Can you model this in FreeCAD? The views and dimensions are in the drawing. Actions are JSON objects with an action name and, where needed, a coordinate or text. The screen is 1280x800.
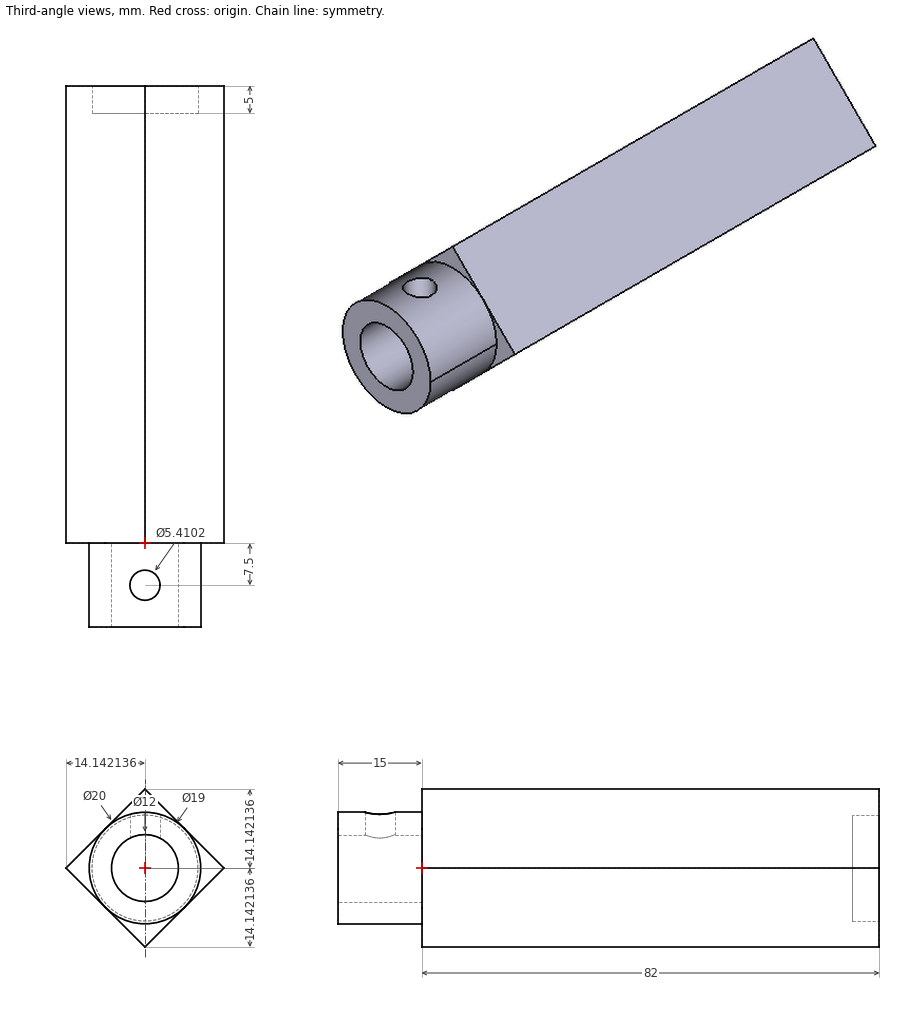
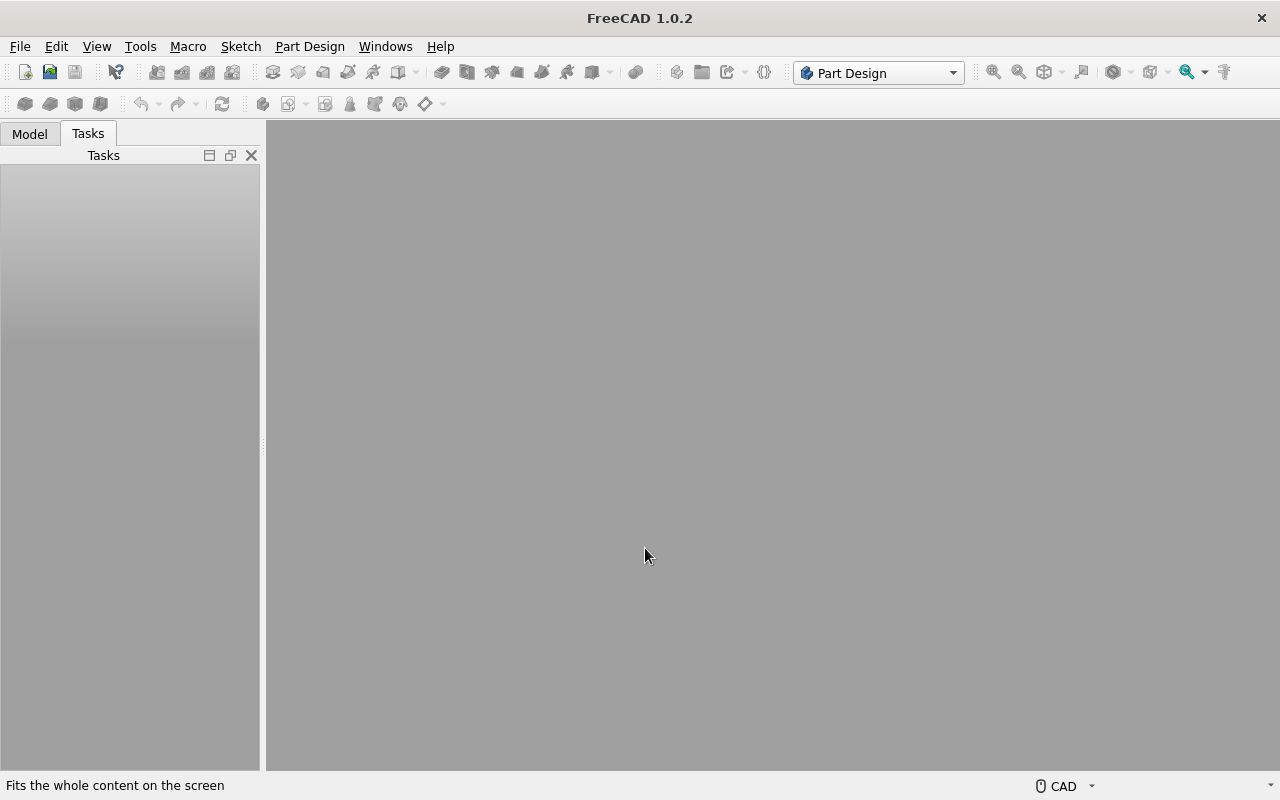
{"action": "left_click", "coordinate": [25, 72]}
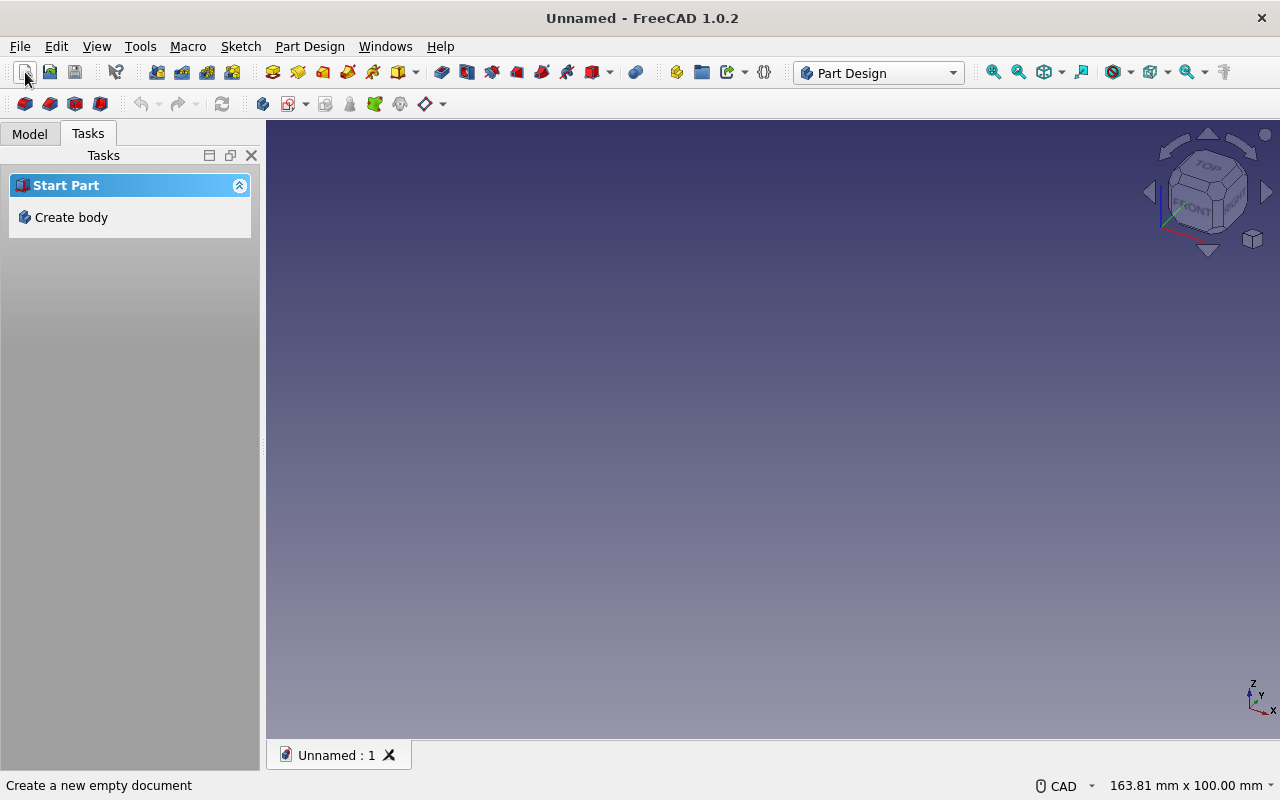
{"action": "left_click", "coordinate": [288, 104]}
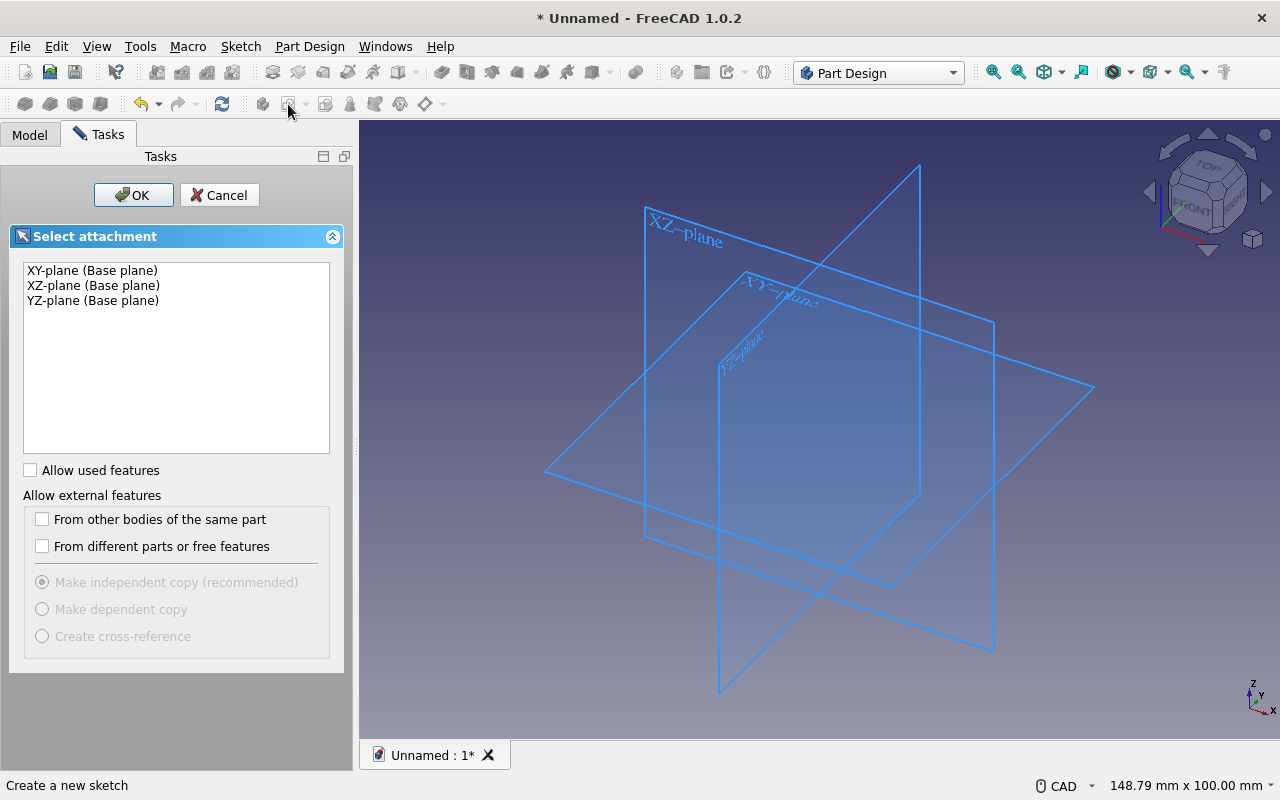
{"action": "left_click", "coordinate": [84, 286]}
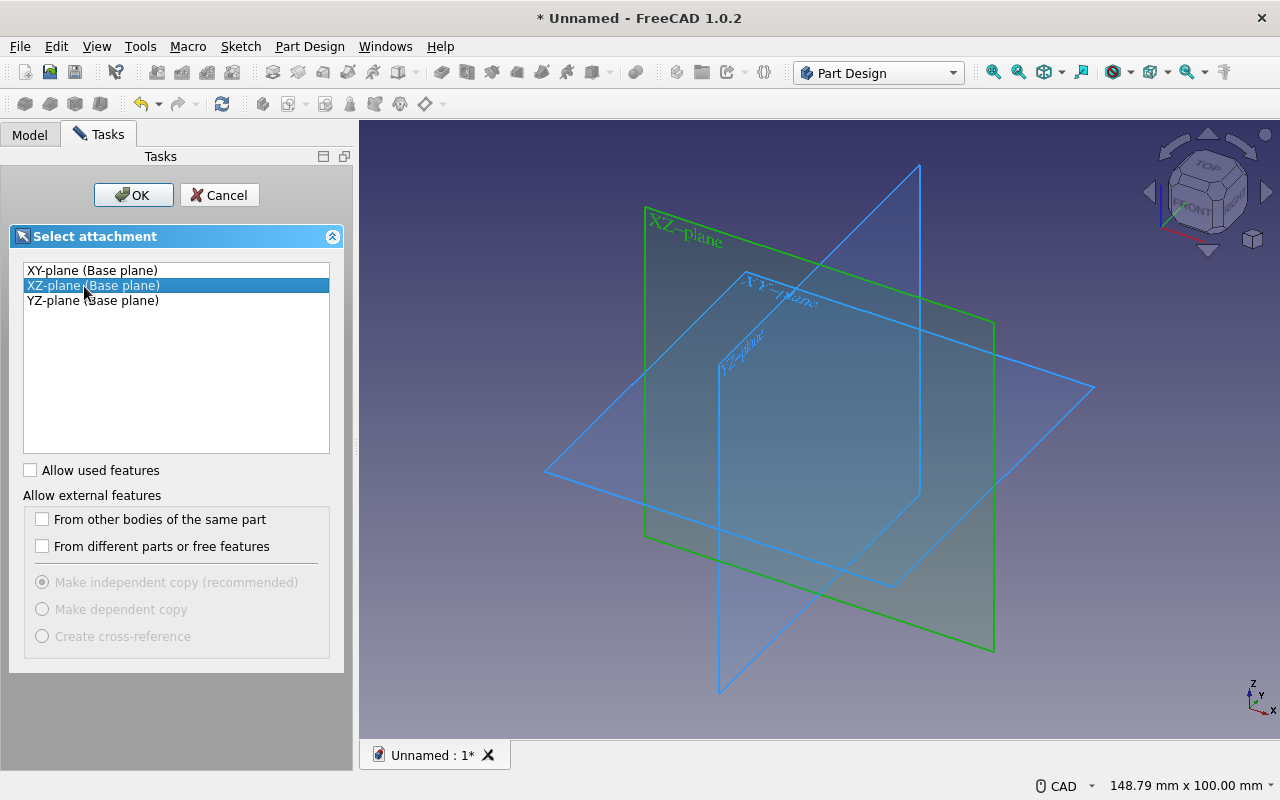
{"action": "left_click", "coordinate": [134, 195]}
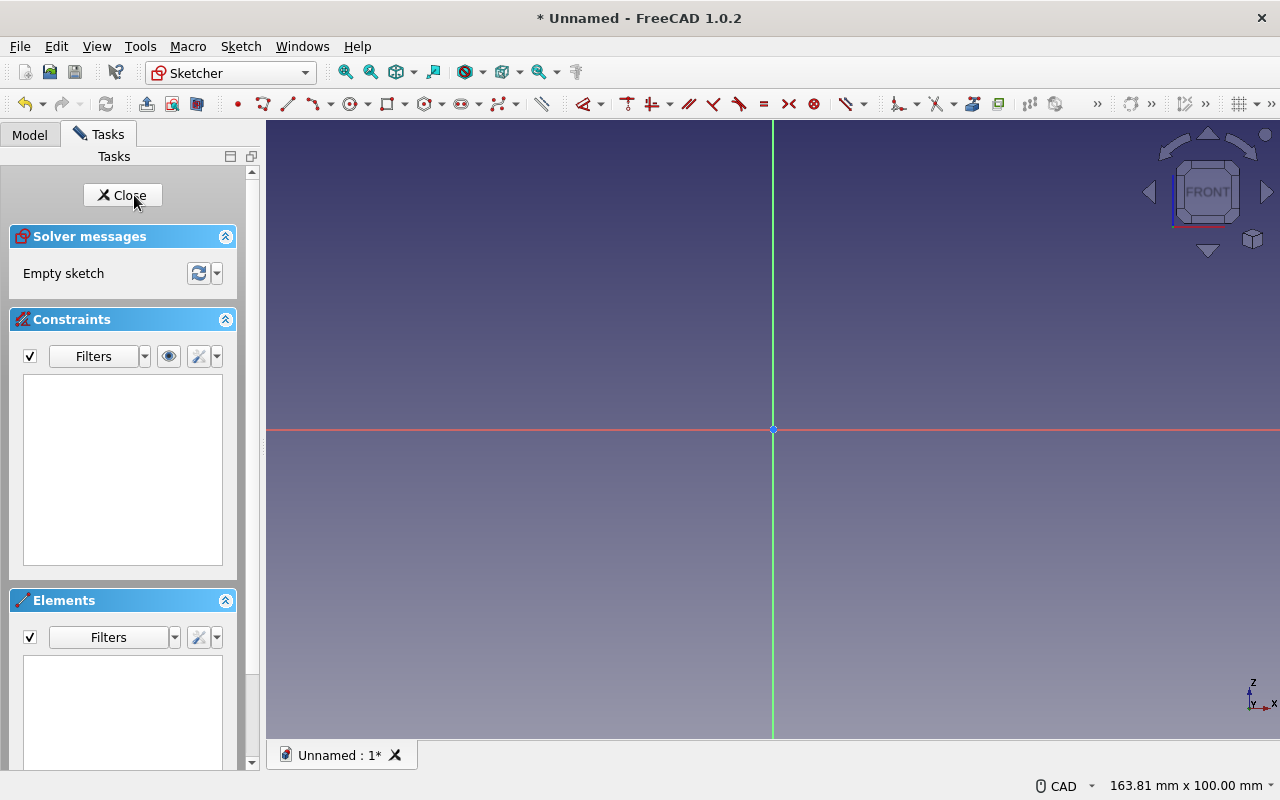
{"action": "scroll", "coordinate": [829, 430], "scroll_direction": "up", "scroll_amount": 4}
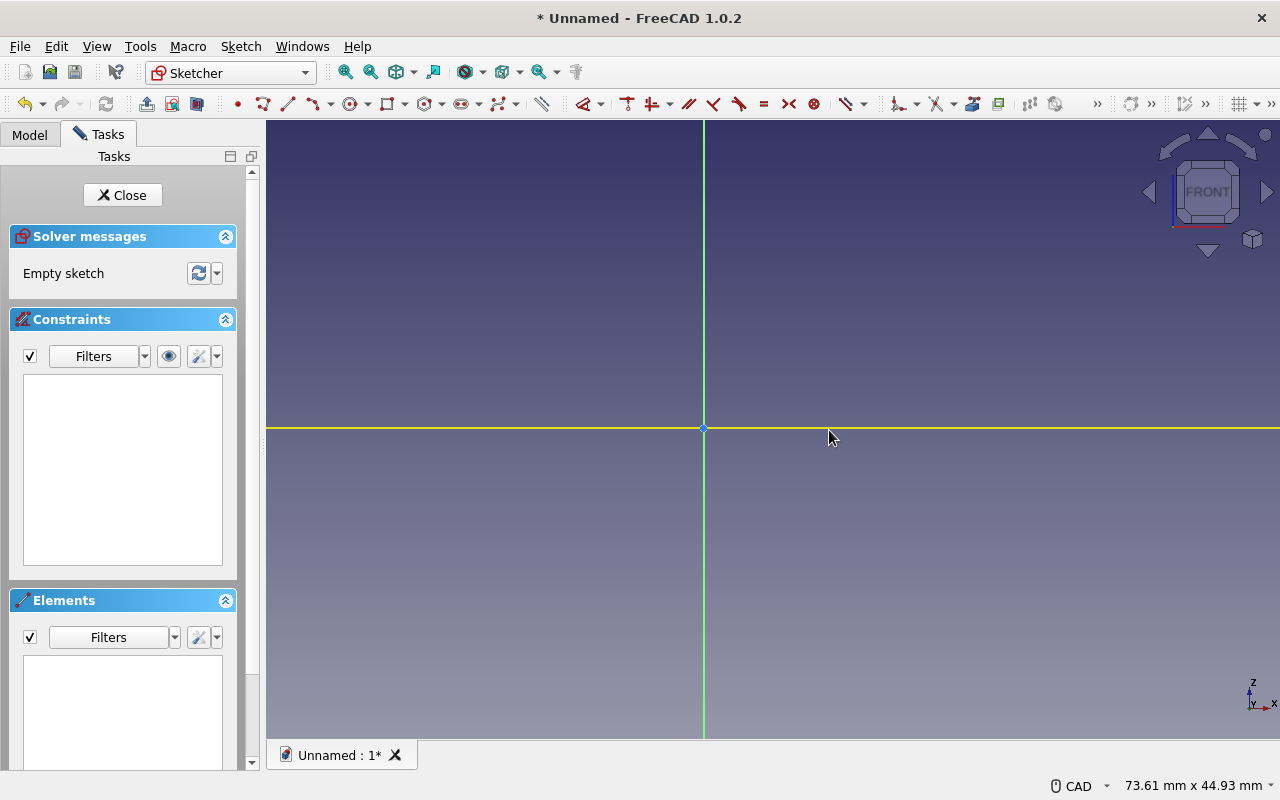
{"action": "key", "text": "g m"}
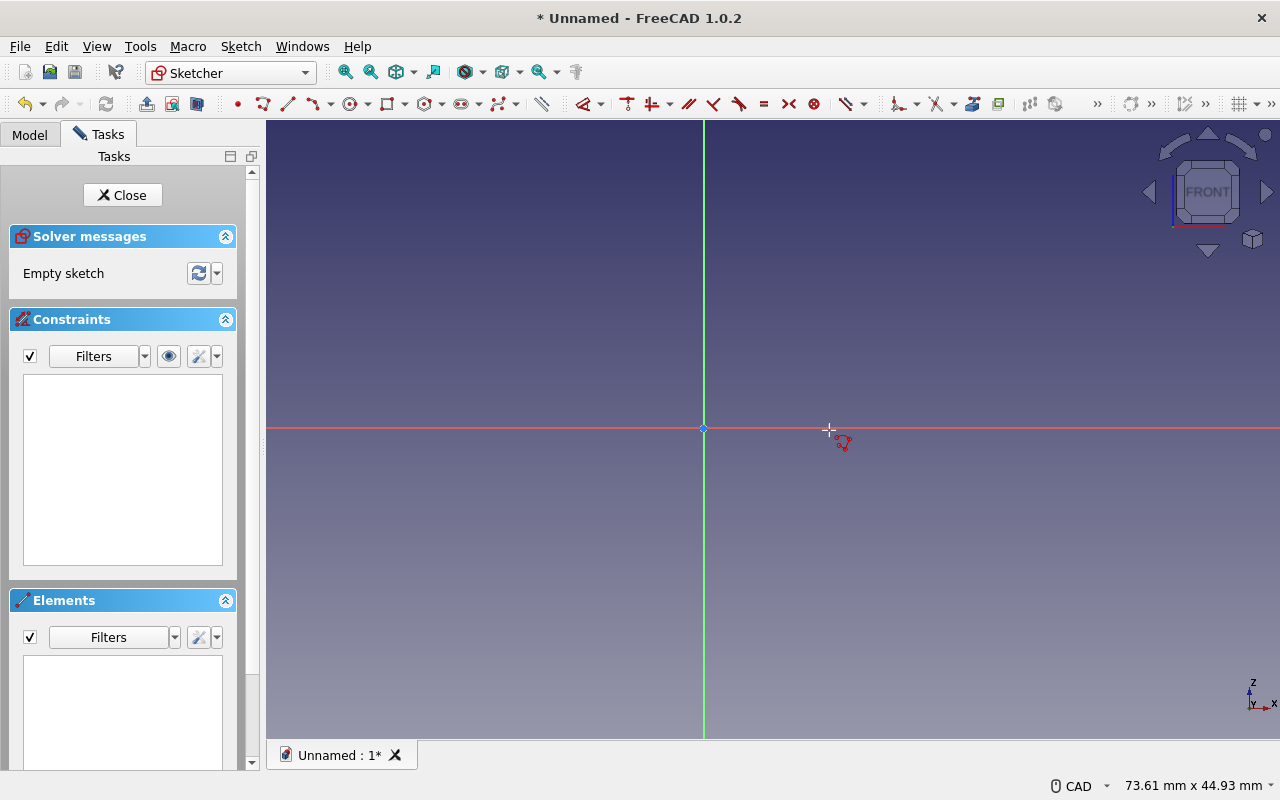
{"action": "left_click", "coordinate": [704, 623]}
{"action": "left_click", "coordinate": [509, 428]}
{"action": "left_click", "coordinate": [704, 233]}
{"action": "left_click", "coordinate": [899, 428]}
{"action": "left_click", "coordinate": [704, 624]}
{"action": "key", "text": "Escape"}
{"action": "key", "text": "Escape"}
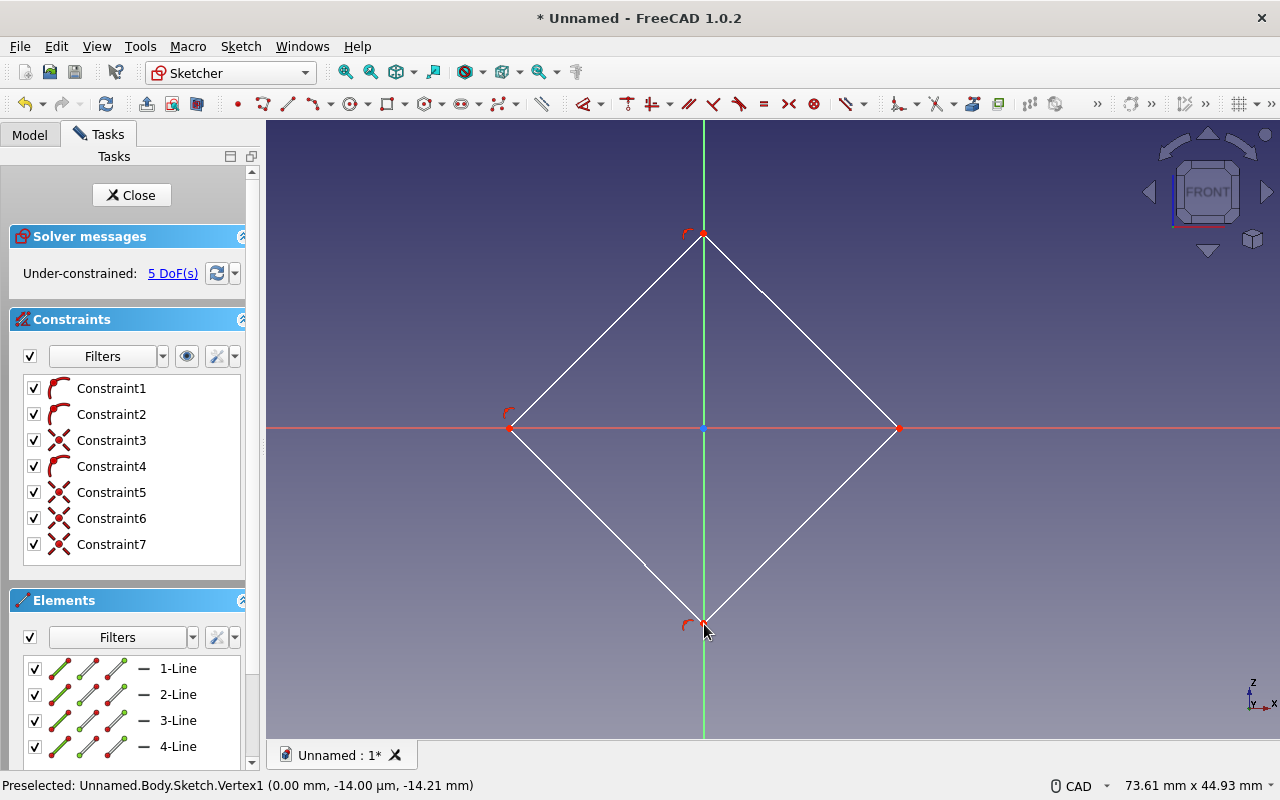
{"action": "left_click", "coordinate": [509, 428]}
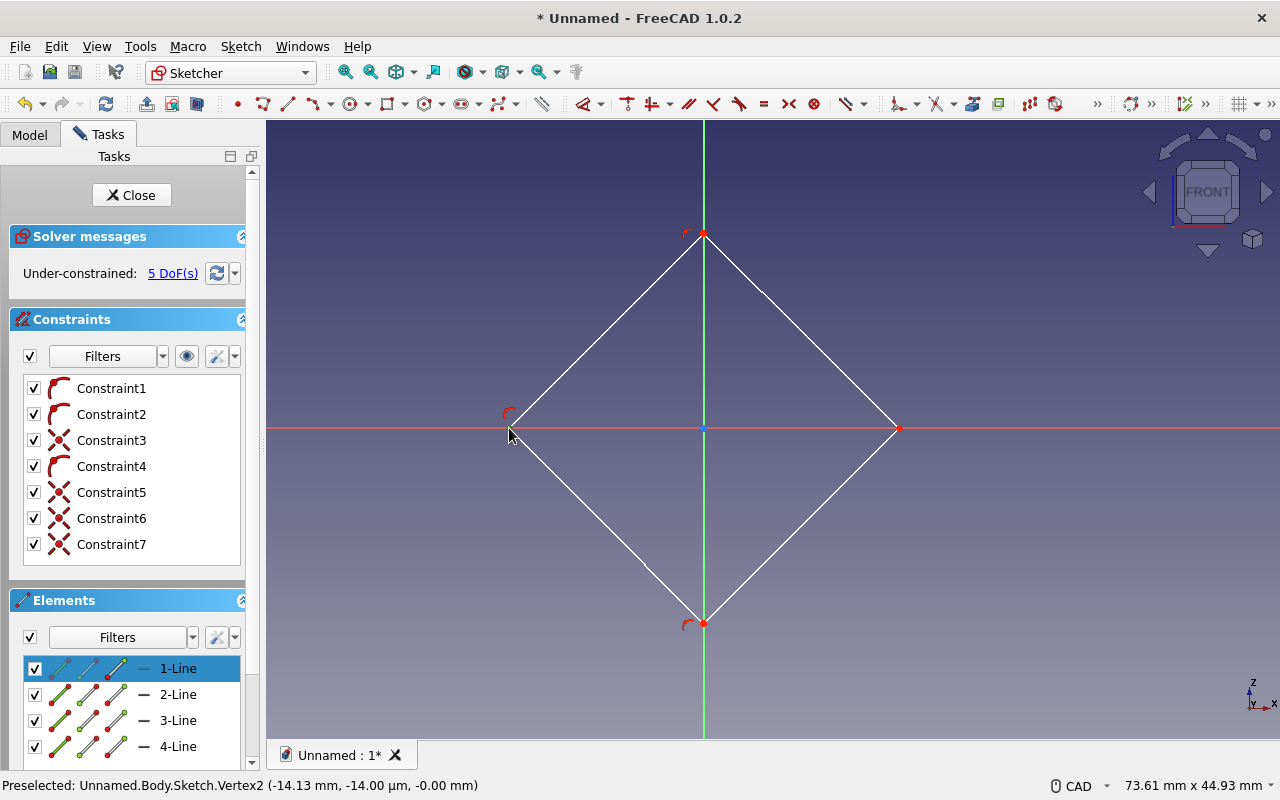
{"action": "left_click", "coordinate": [899, 428]}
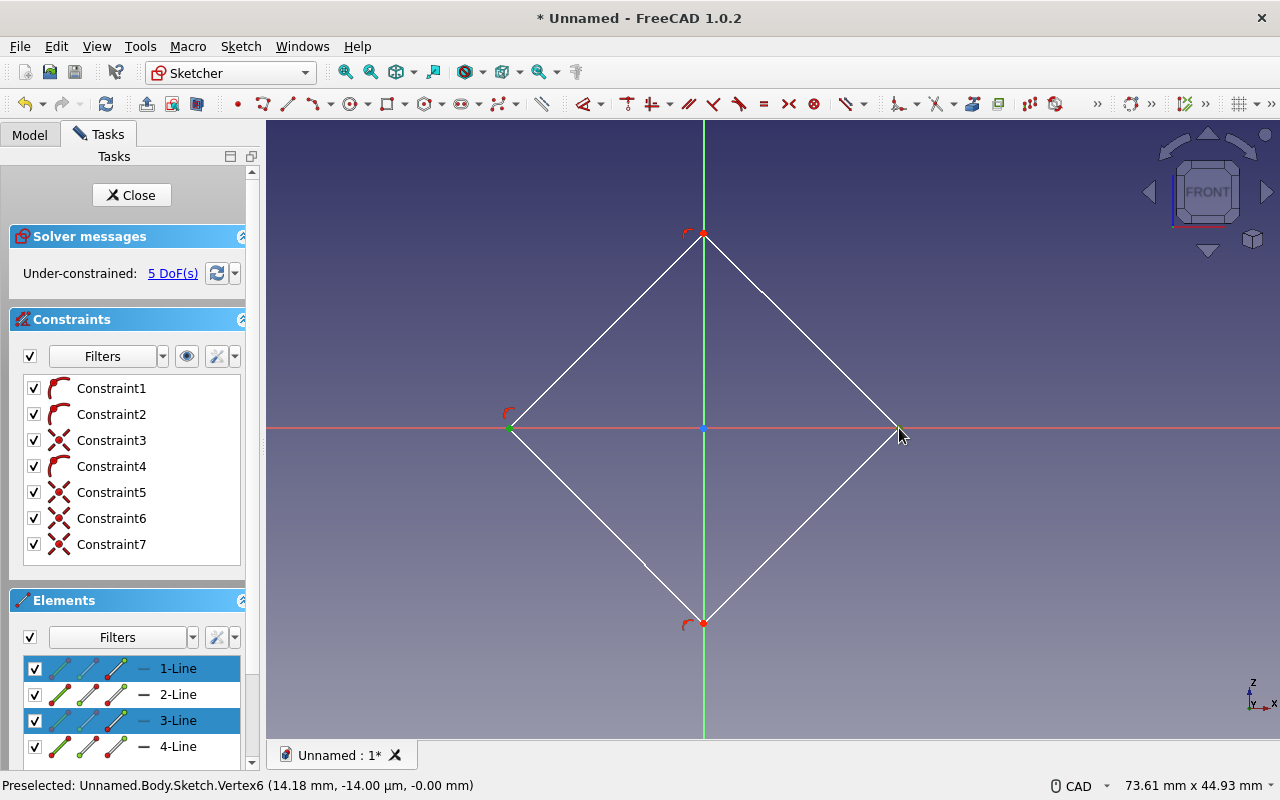
{"action": "left_click", "coordinate": [704, 671]}